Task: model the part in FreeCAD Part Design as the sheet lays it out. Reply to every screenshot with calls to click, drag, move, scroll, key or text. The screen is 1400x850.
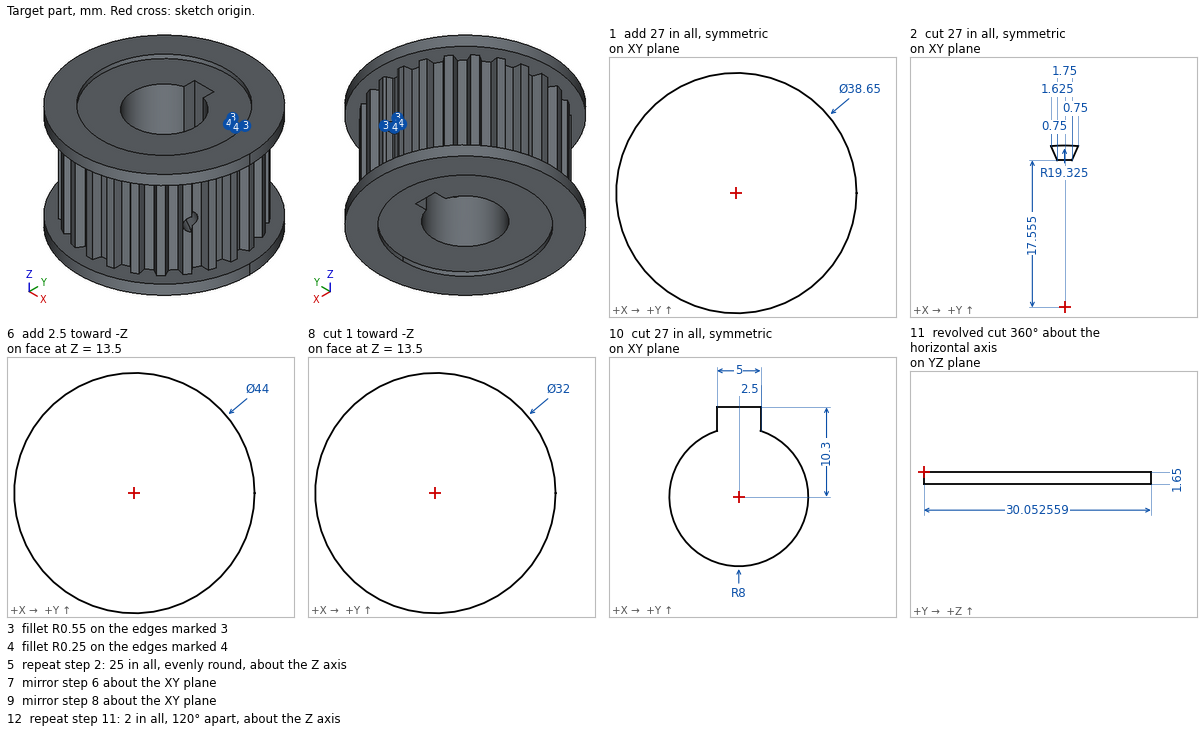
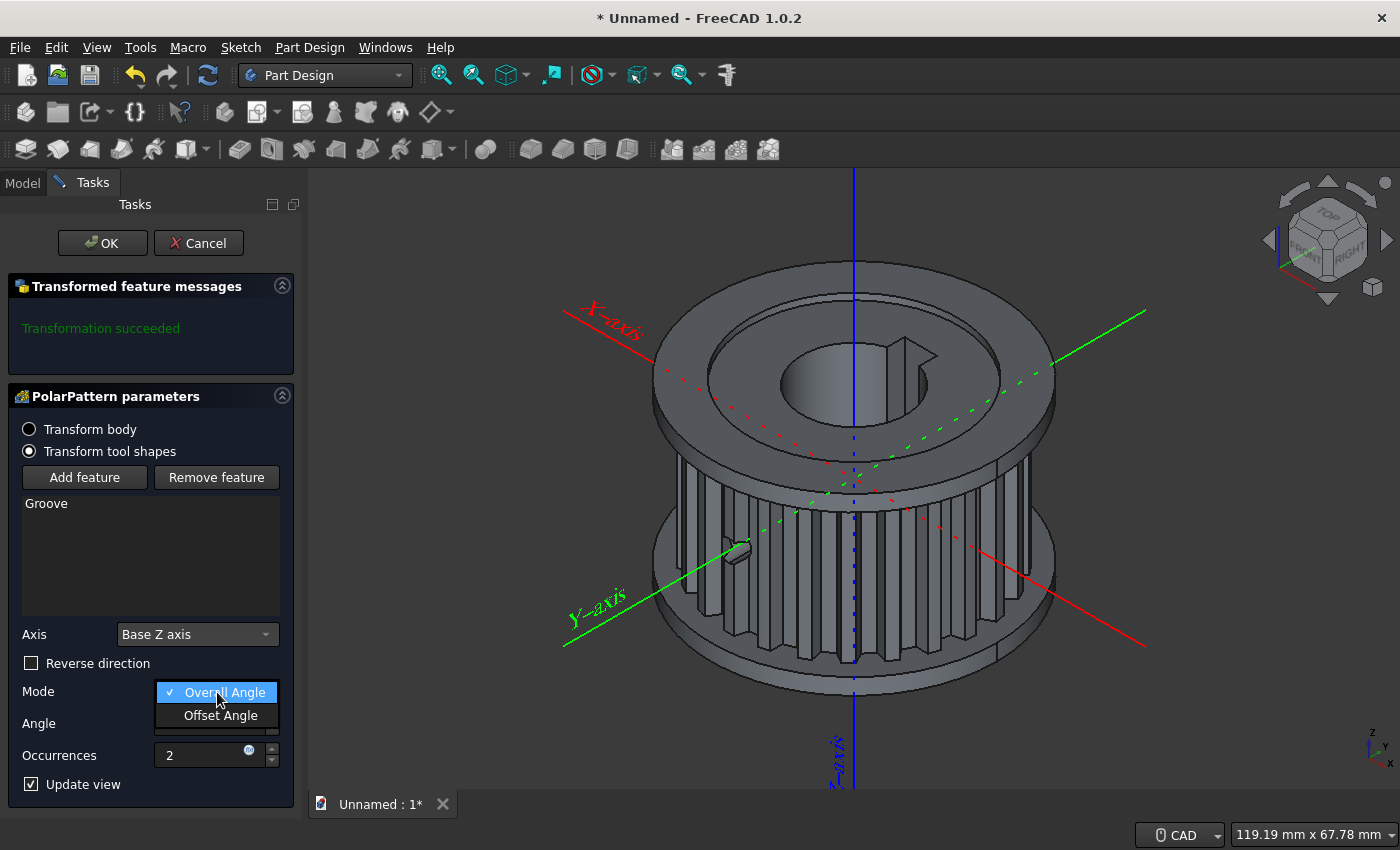
click(216, 716)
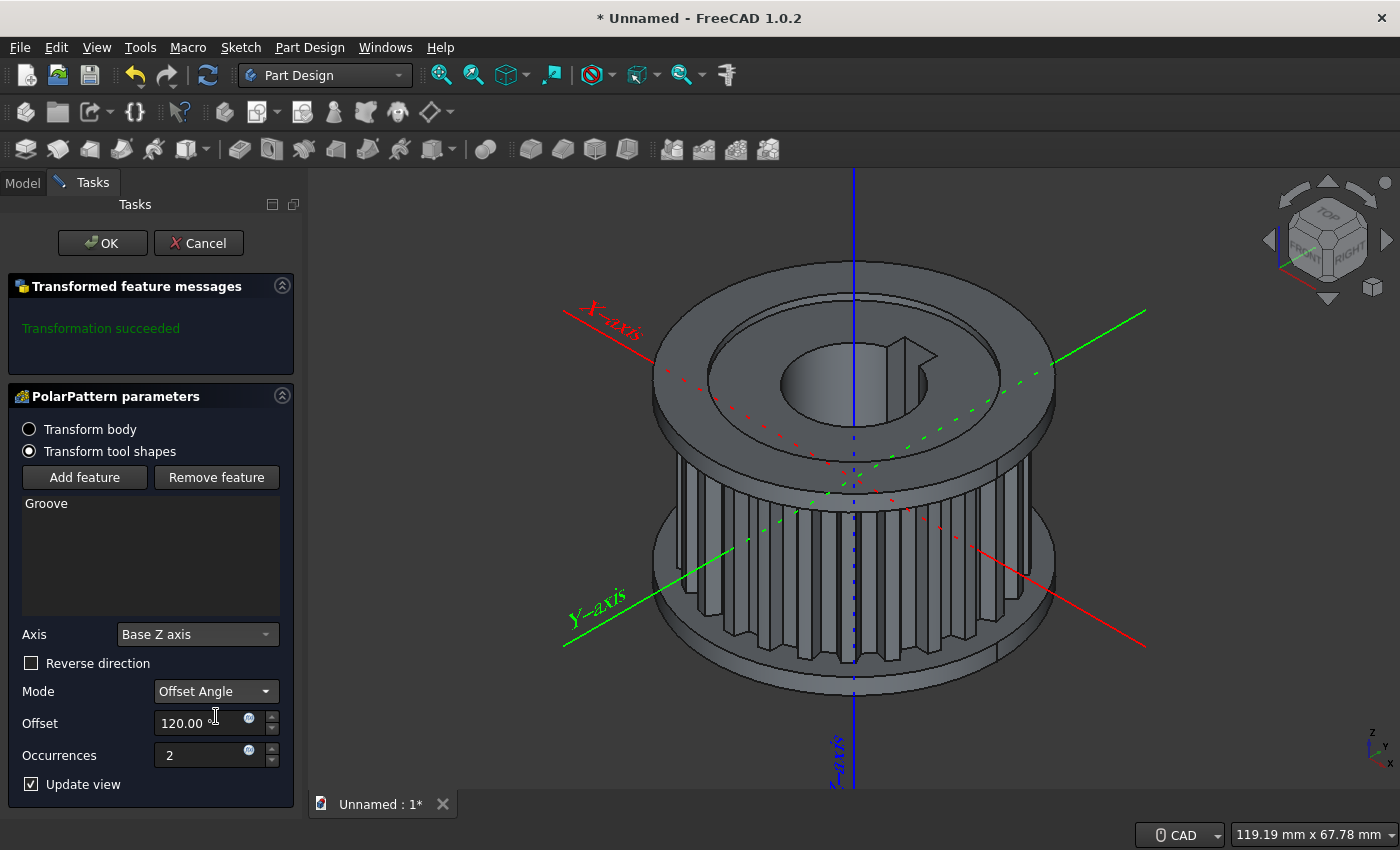
triple_click(209, 723)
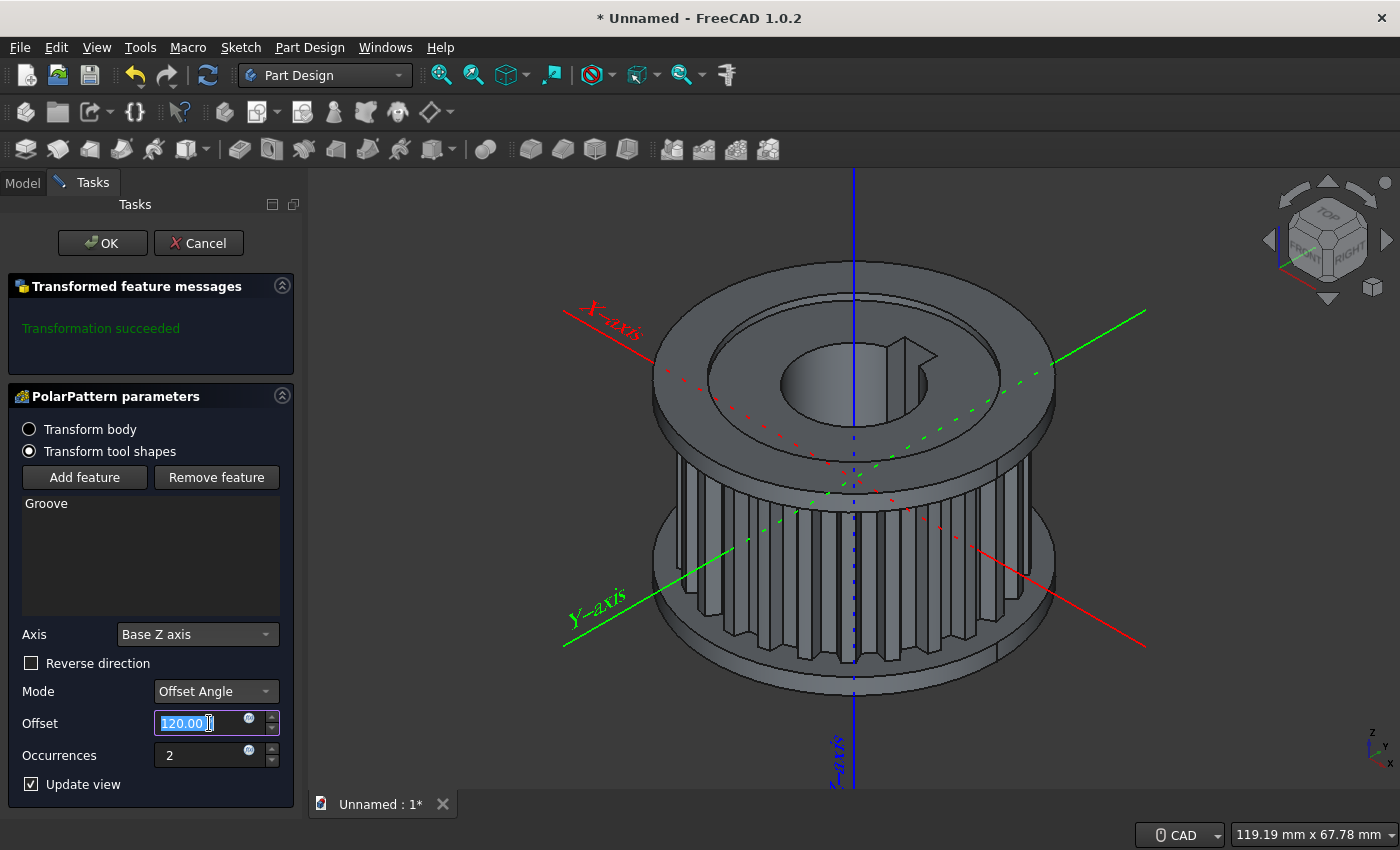
text(120)
key(Tab)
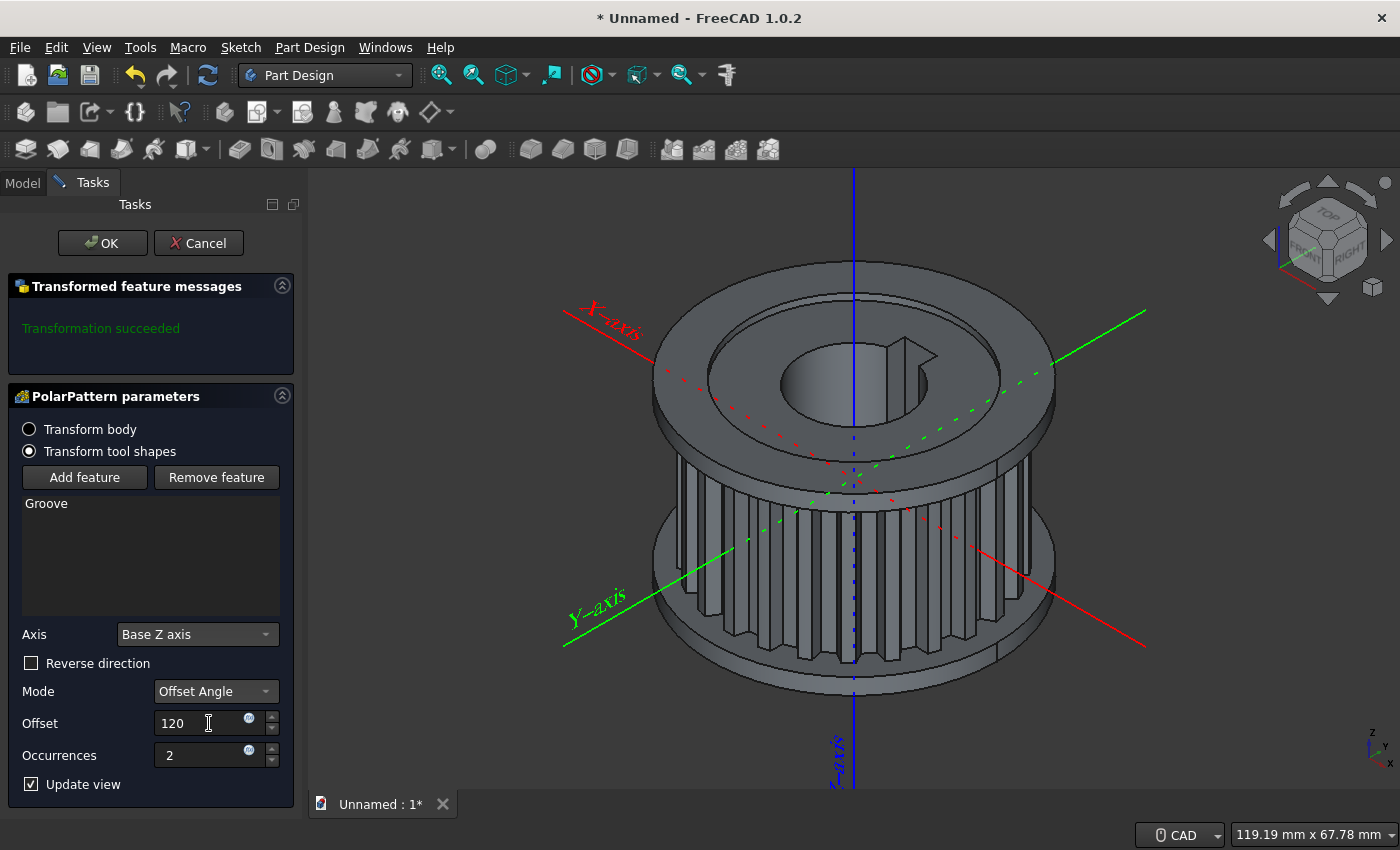
triple_click(209, 755)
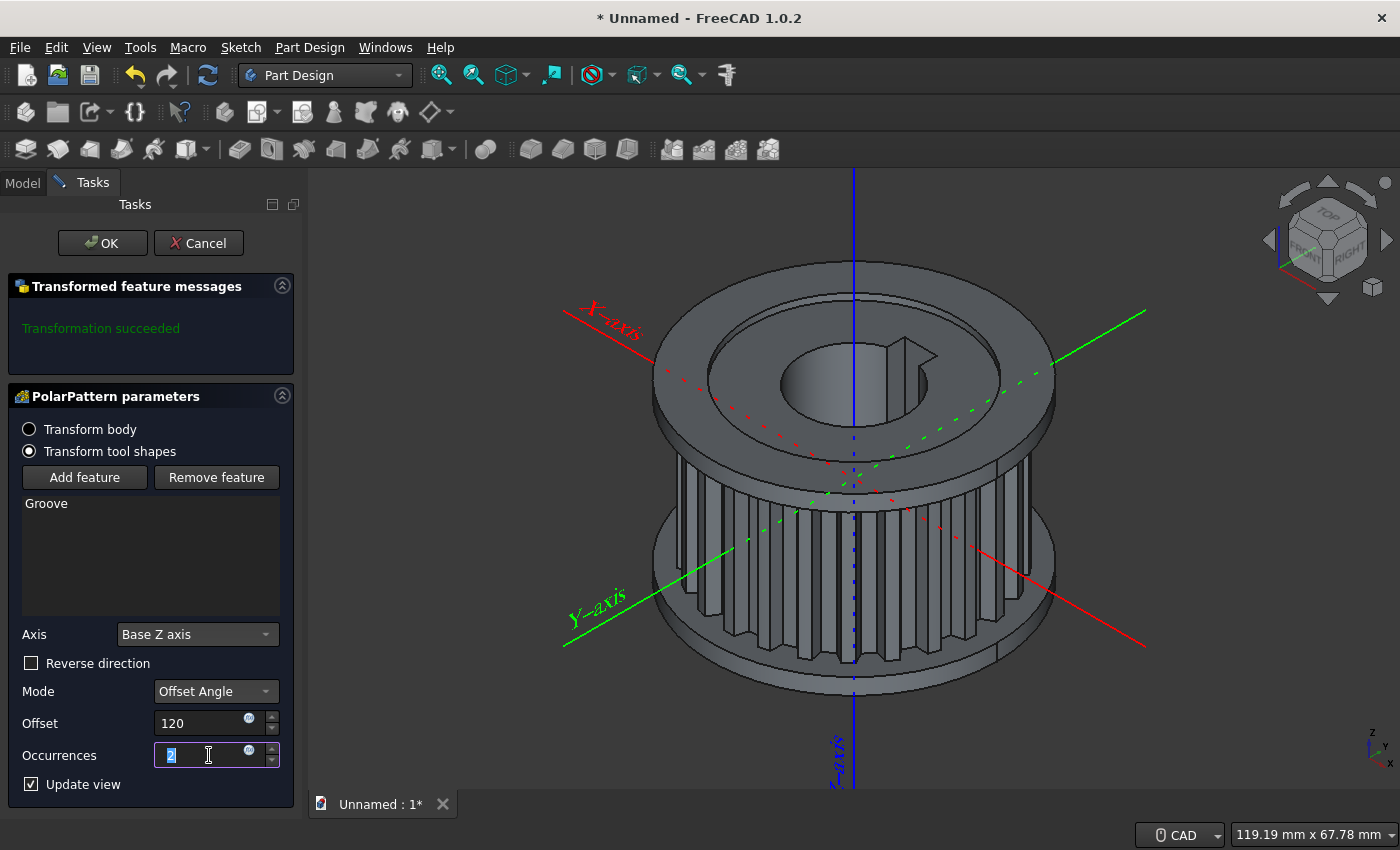
text(2)
key(Tab)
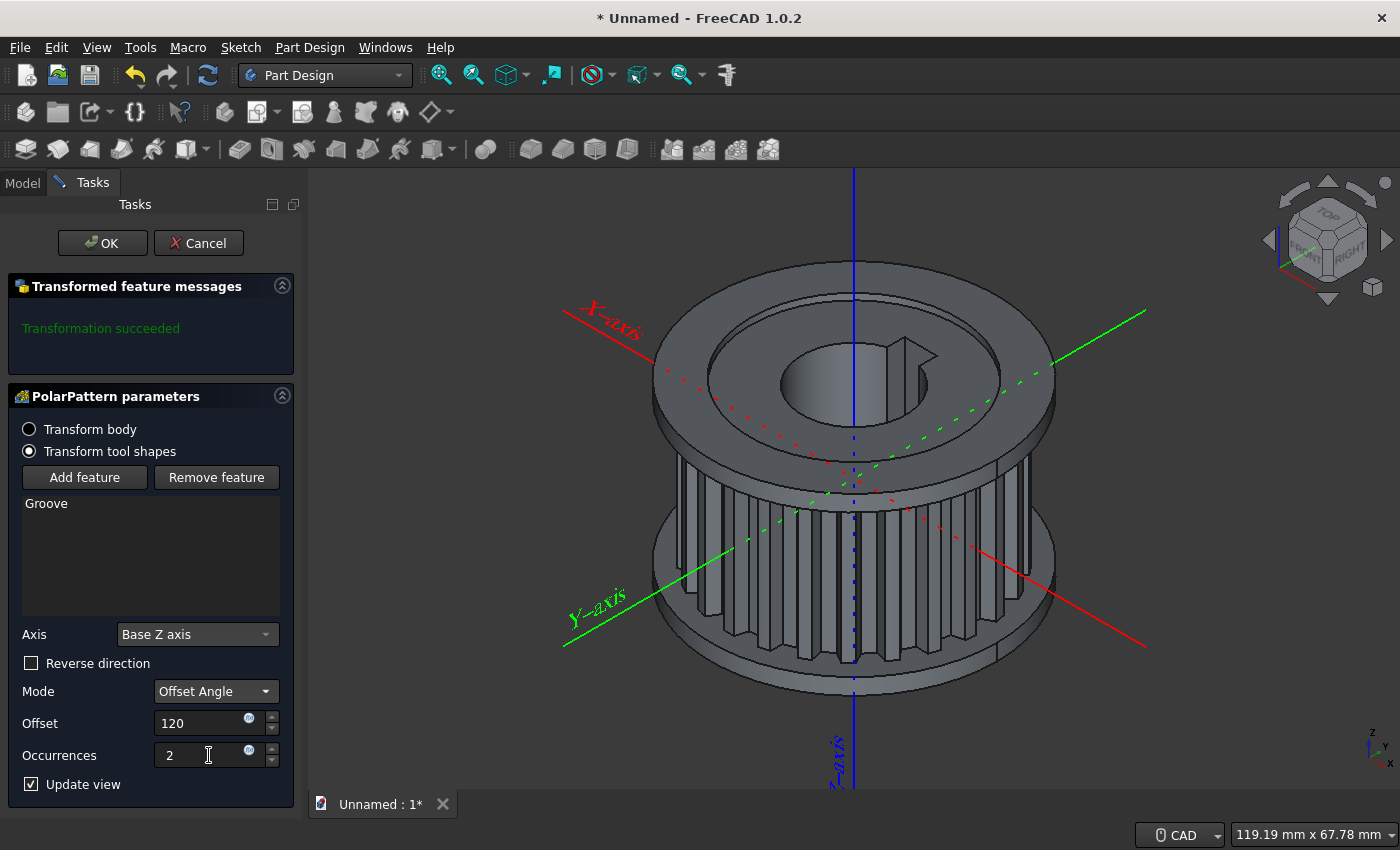
click(30, 663)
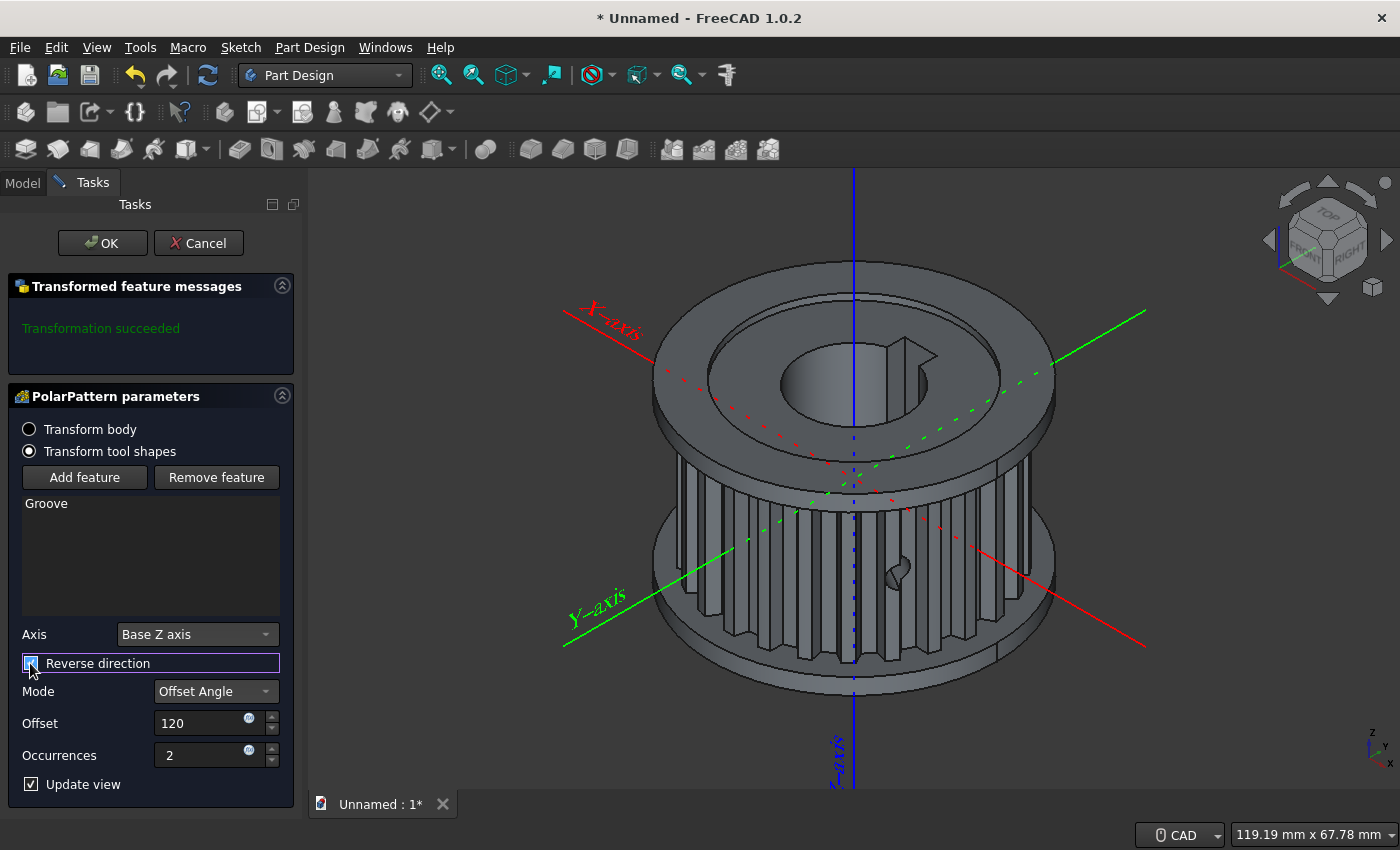
click(103, 243)